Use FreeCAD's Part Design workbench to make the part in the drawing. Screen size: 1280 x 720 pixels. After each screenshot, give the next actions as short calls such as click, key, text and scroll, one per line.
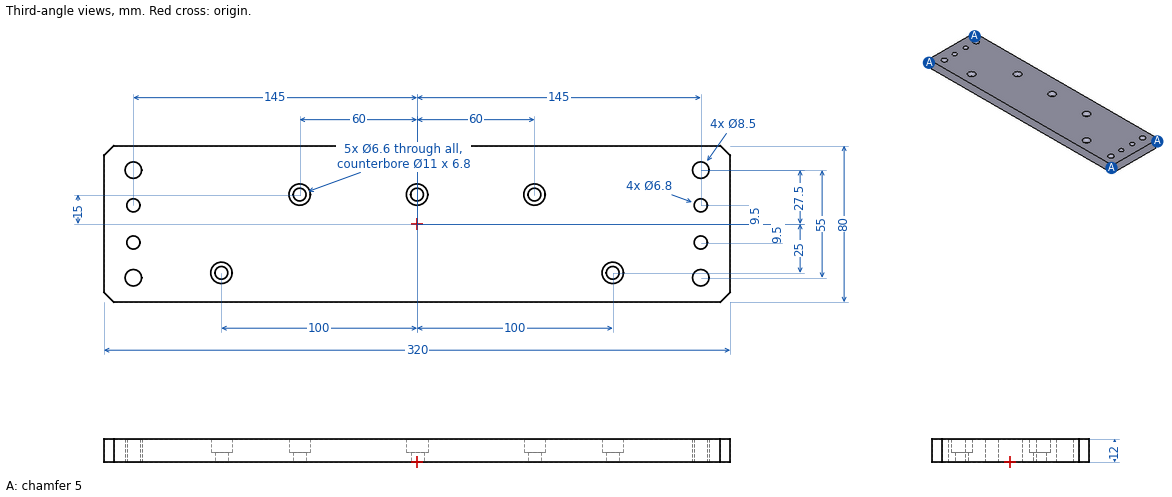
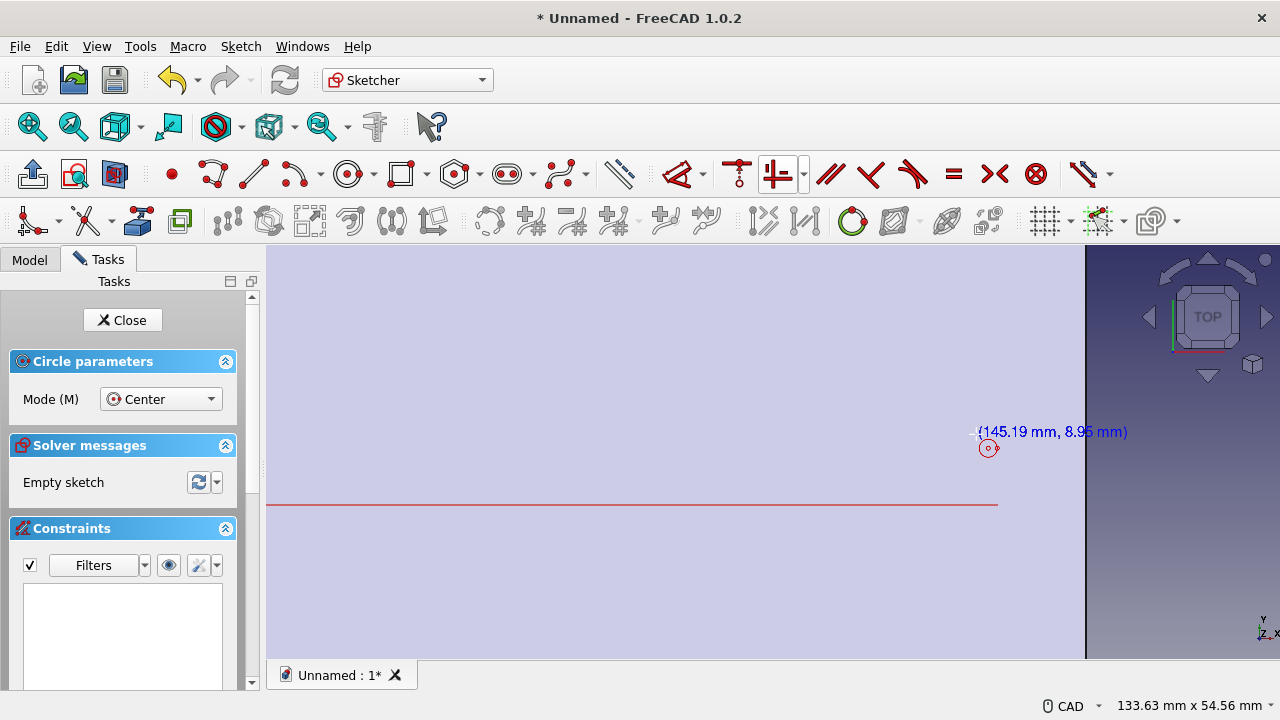
scroll(977, 435, down, 7)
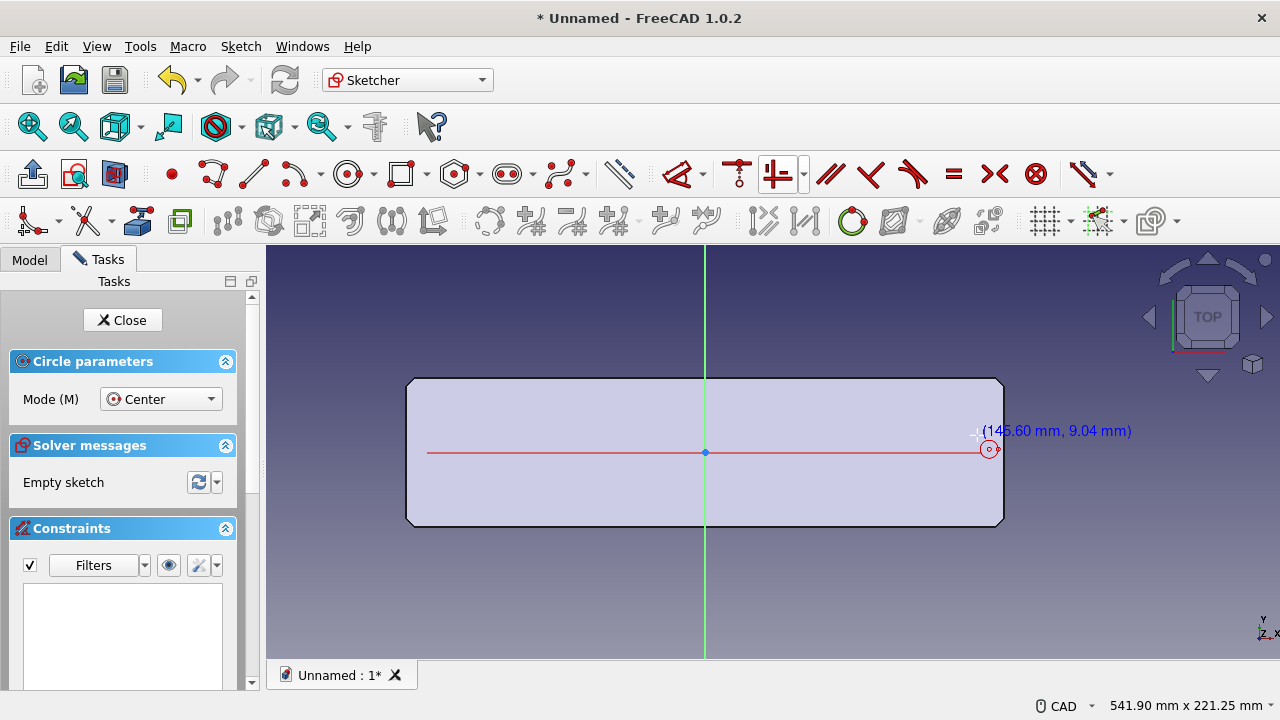
click(976, 435)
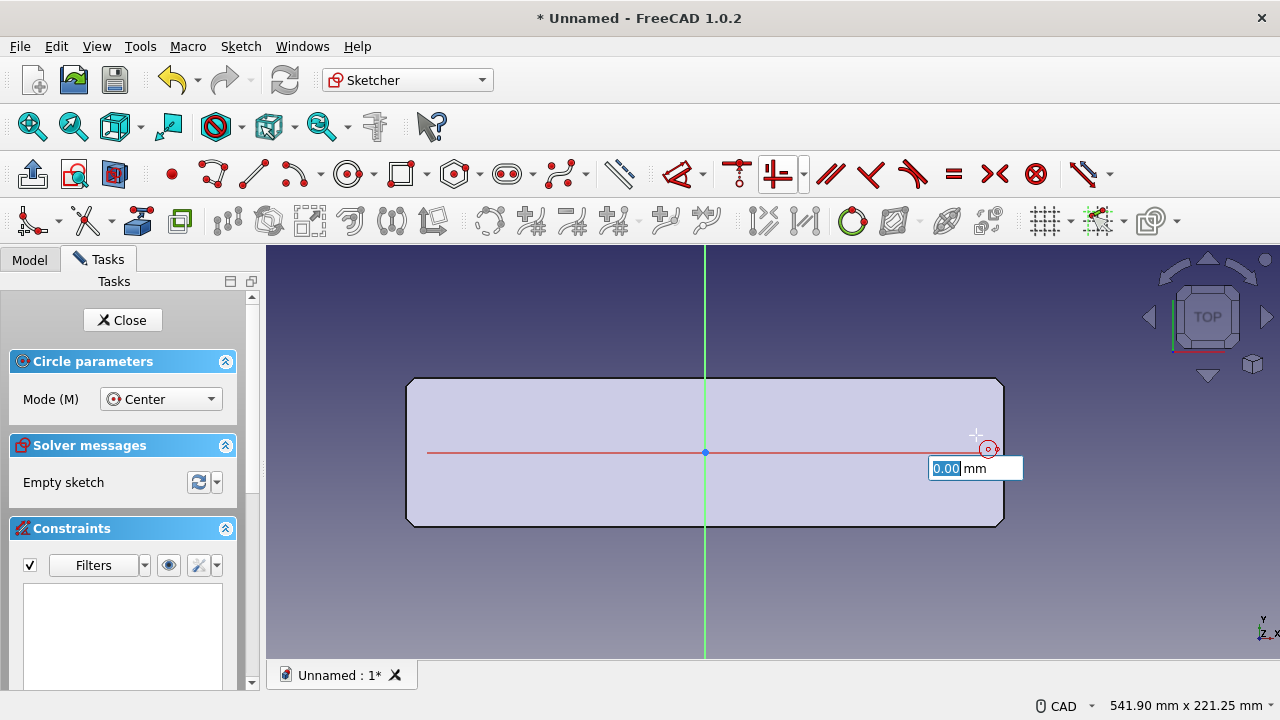
scroll(981, 430, up, 5)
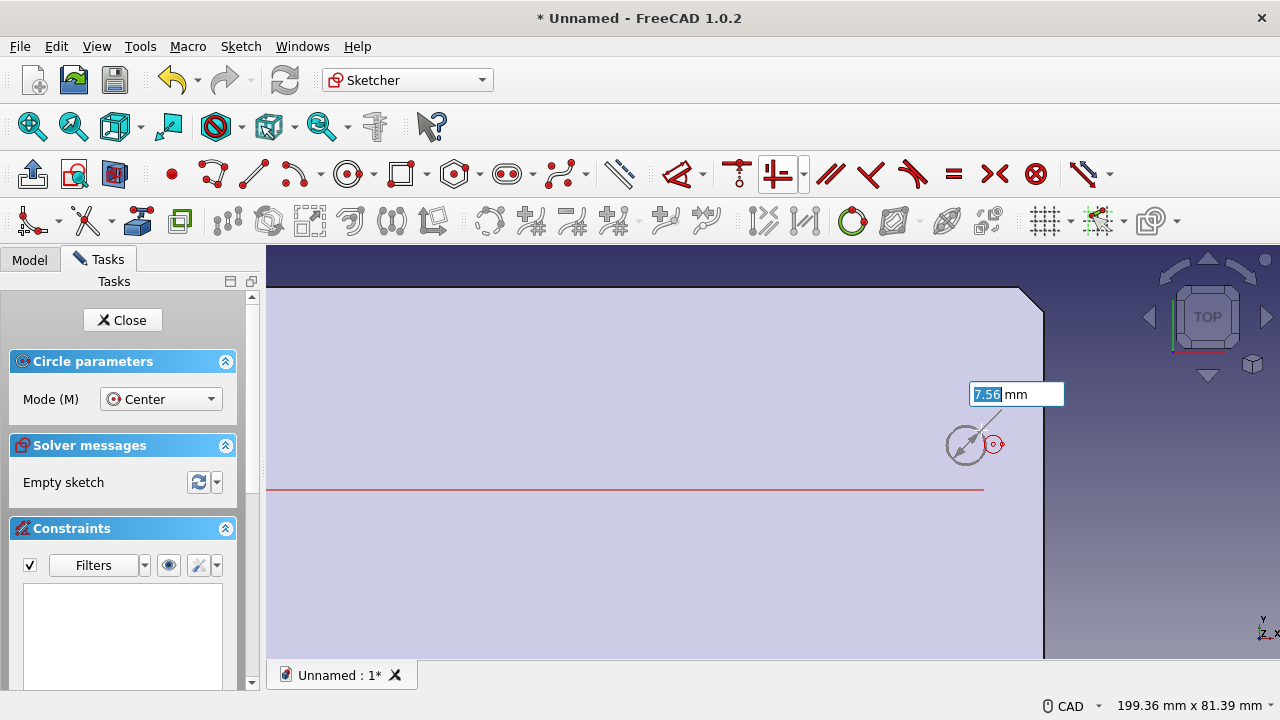
click(980, 430)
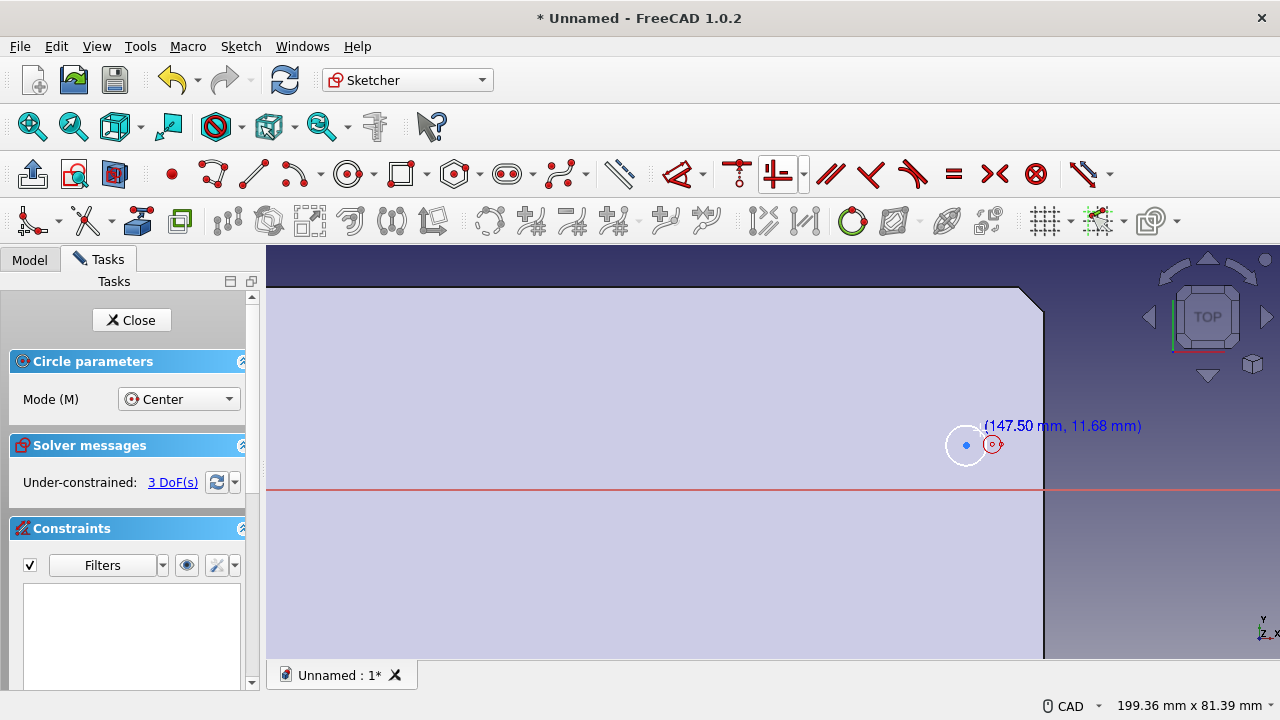
scroll(967, 539, up, 2)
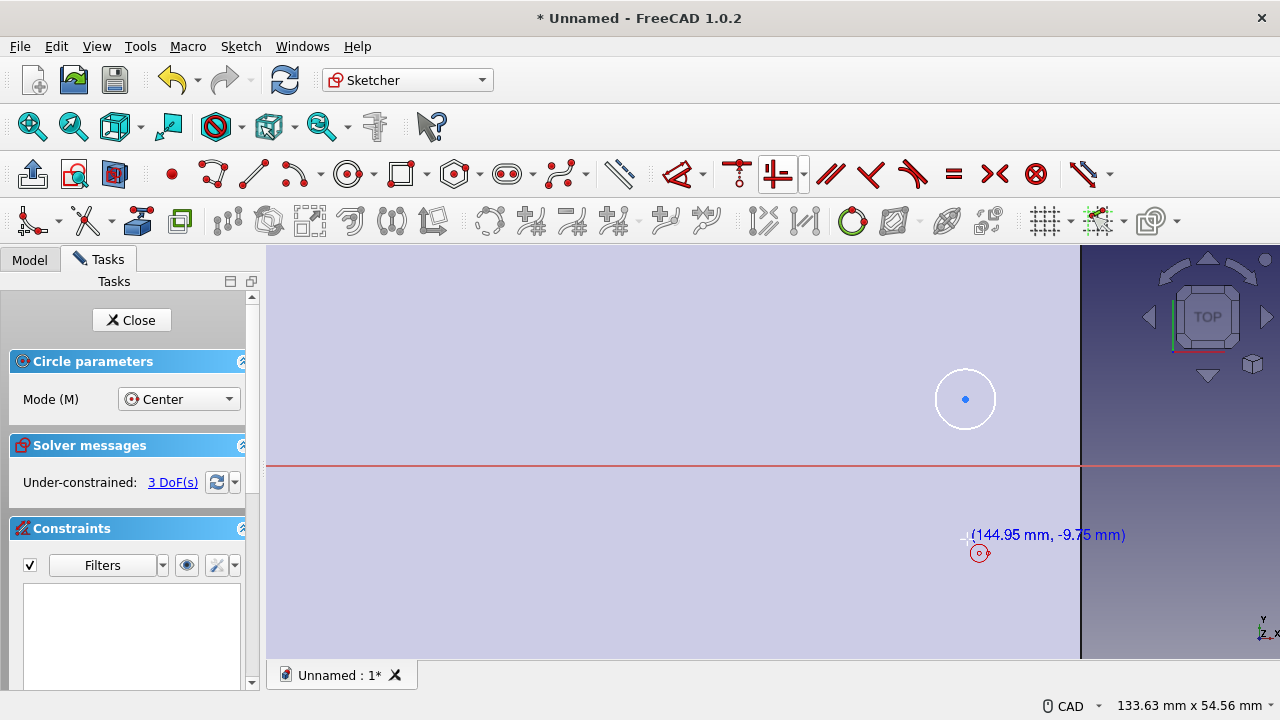
scroll(979, 447, down, 7)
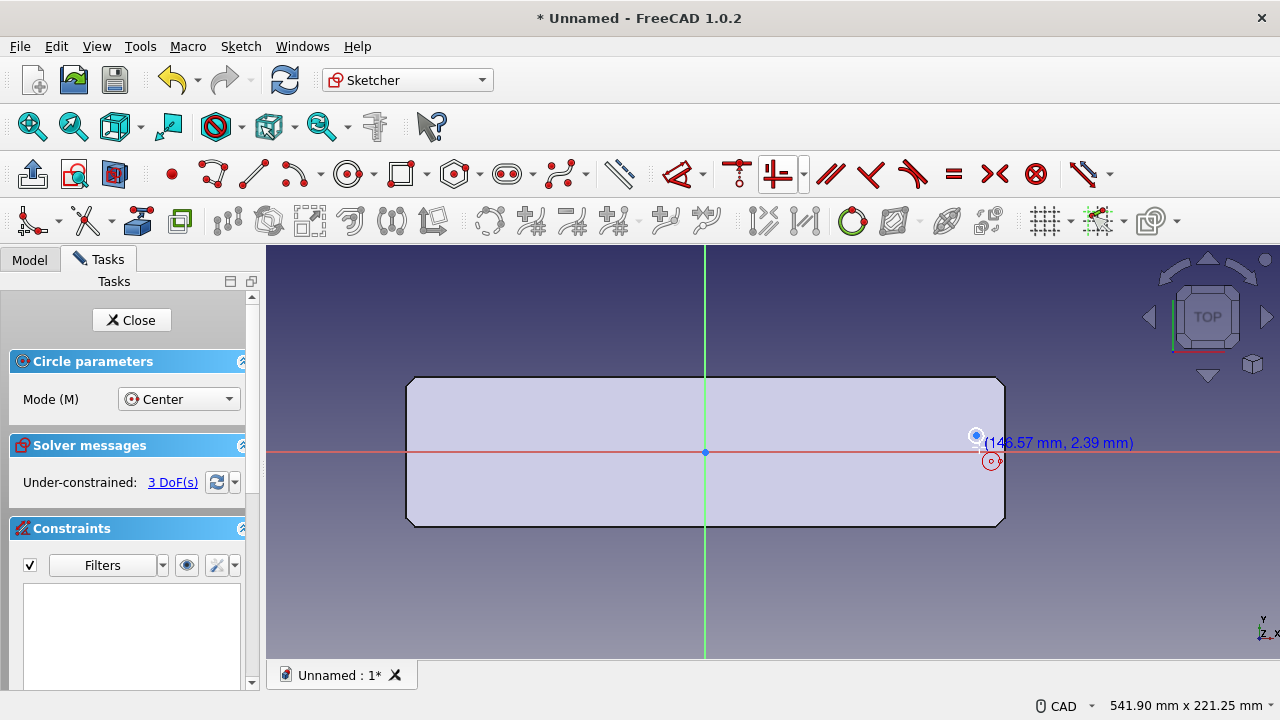
click(977, 470)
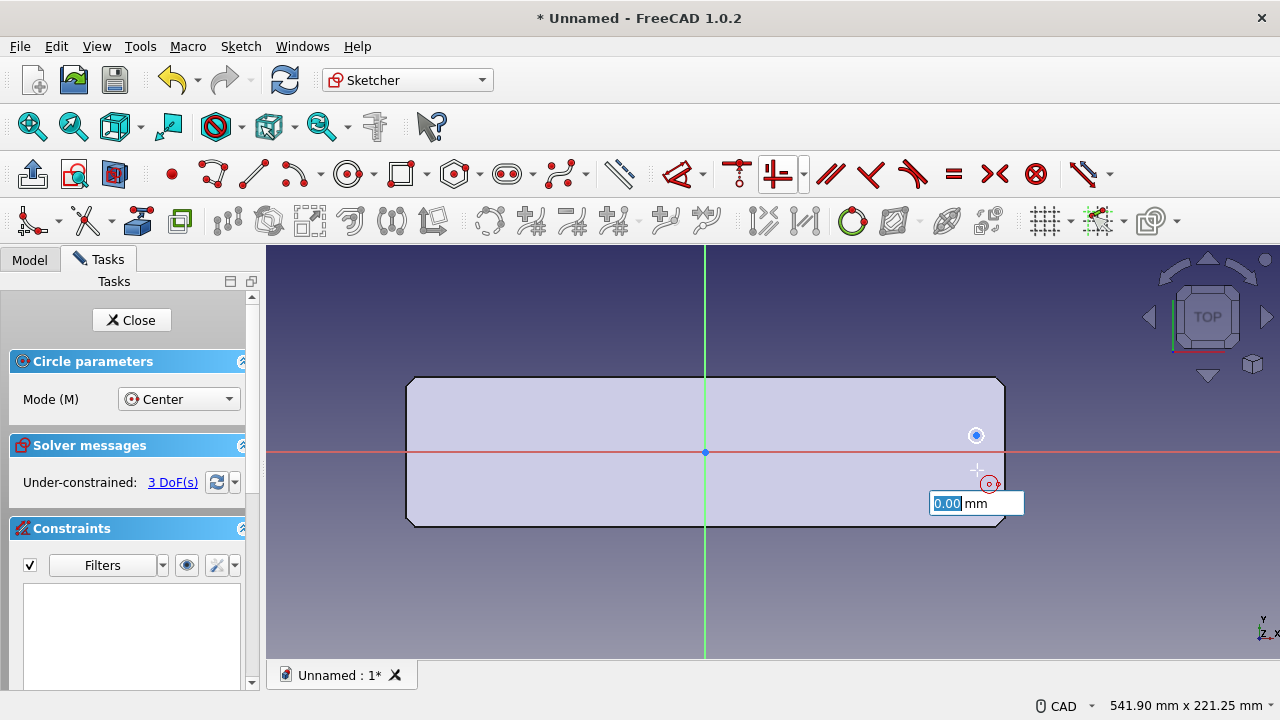
scroll(981, 474, up, 5)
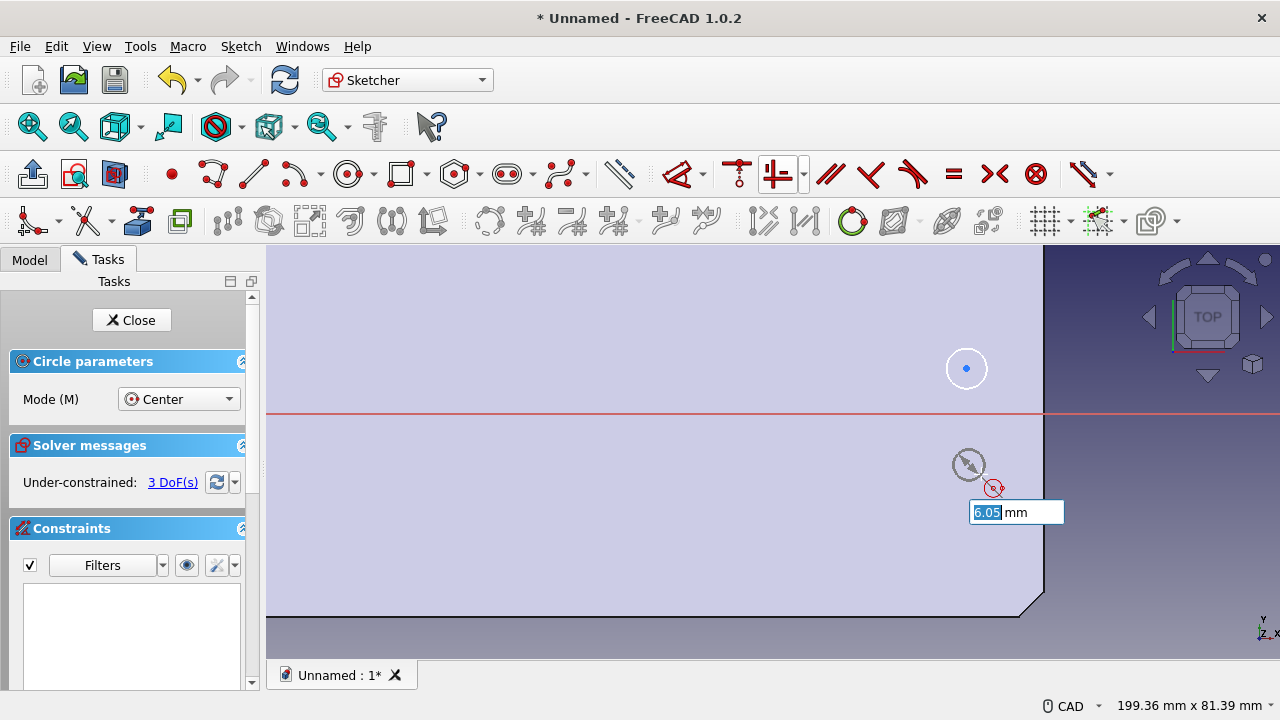
click(980, 474)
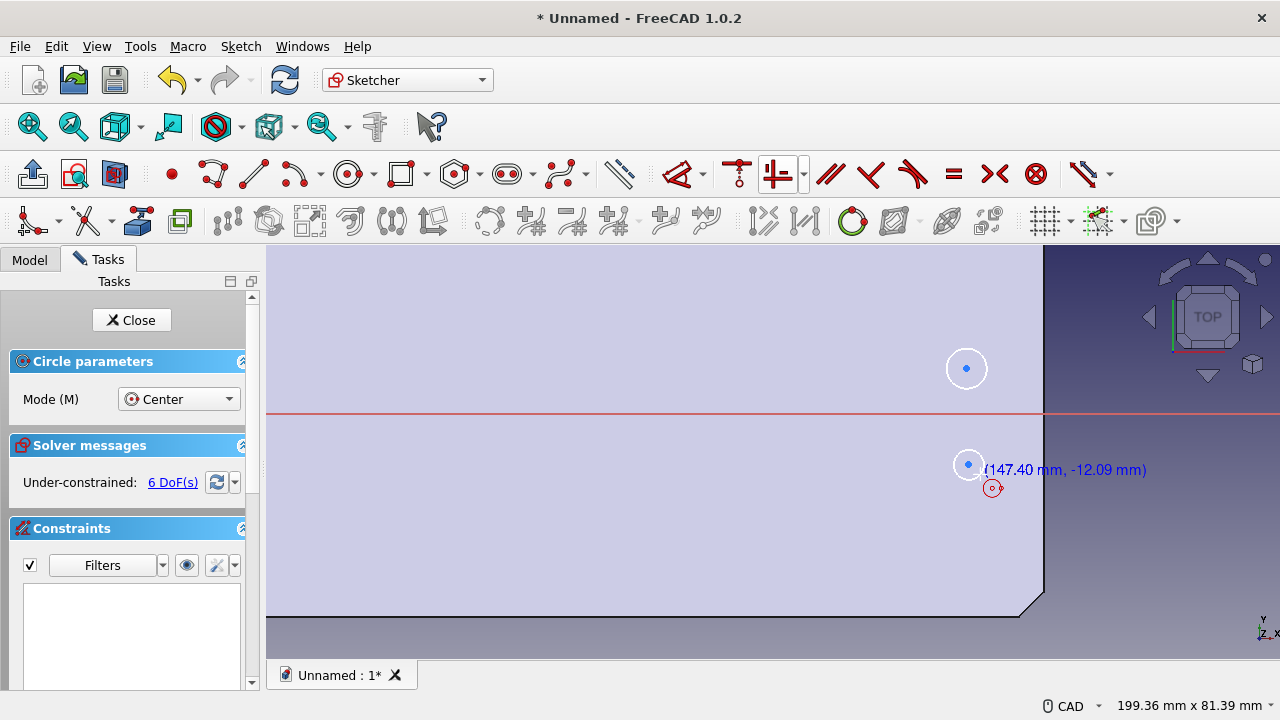
scroll(980, 474, down, 5)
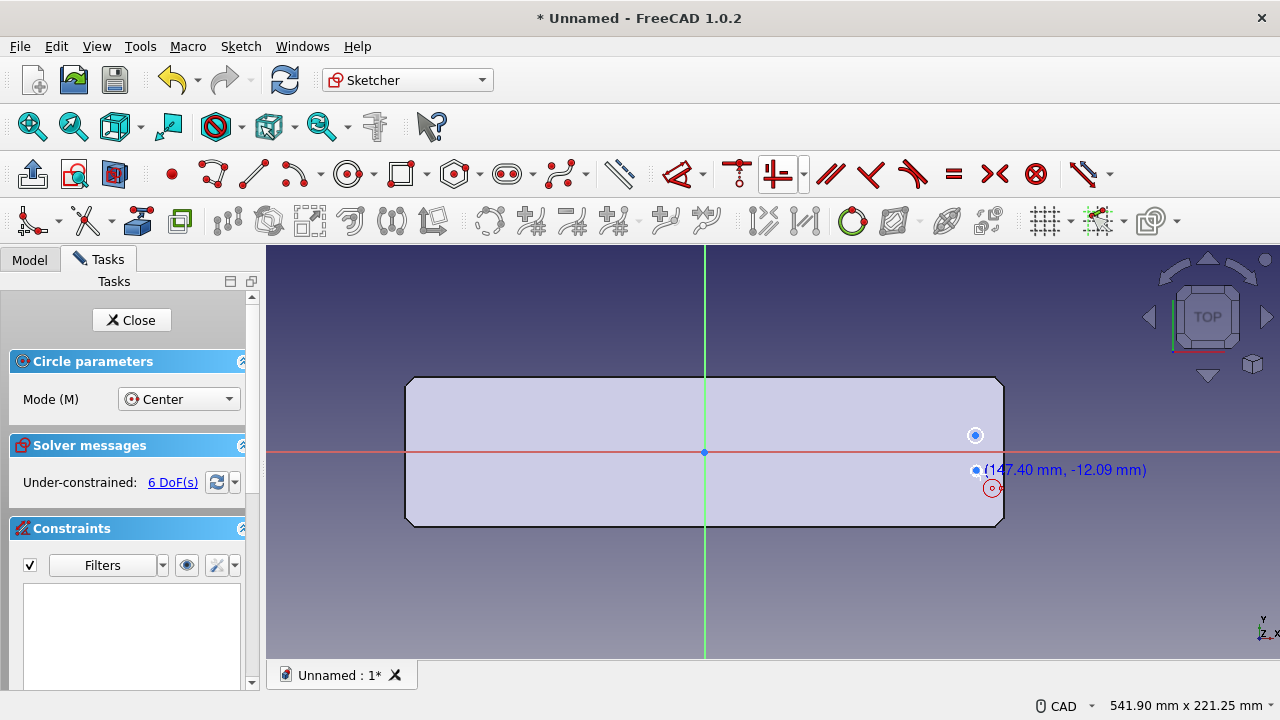
scroll(433, 434, up, 7)